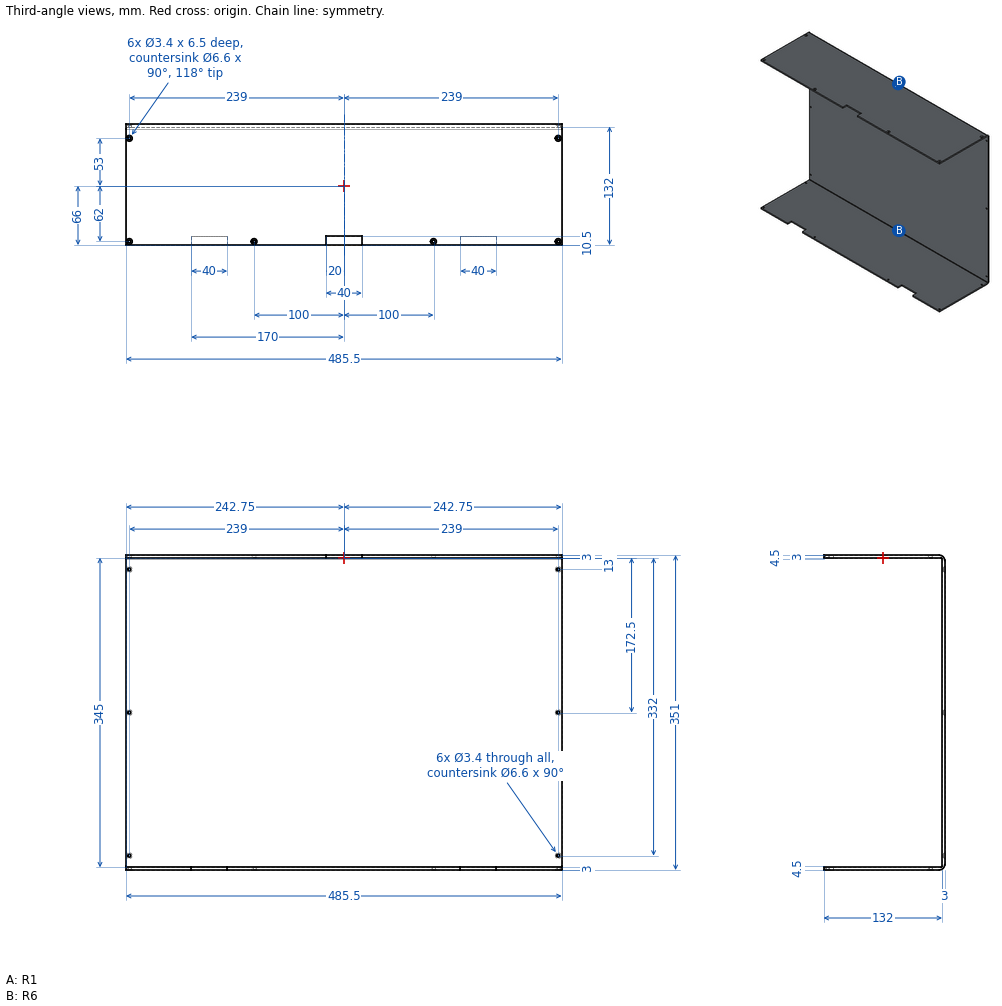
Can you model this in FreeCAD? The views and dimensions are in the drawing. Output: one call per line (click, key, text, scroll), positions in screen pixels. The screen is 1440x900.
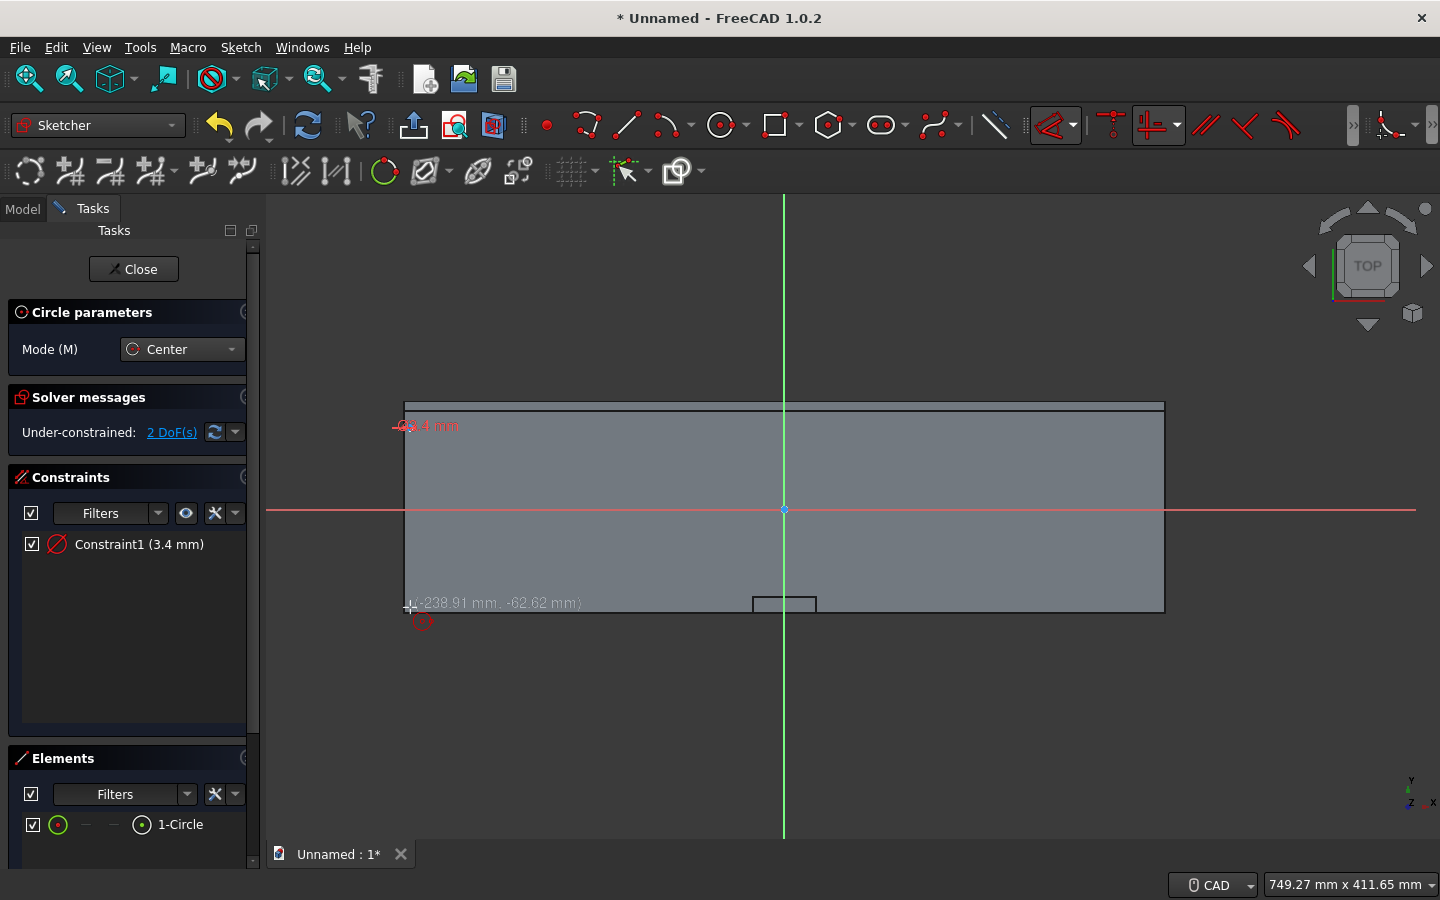
click(410, 607)
move(412, 605)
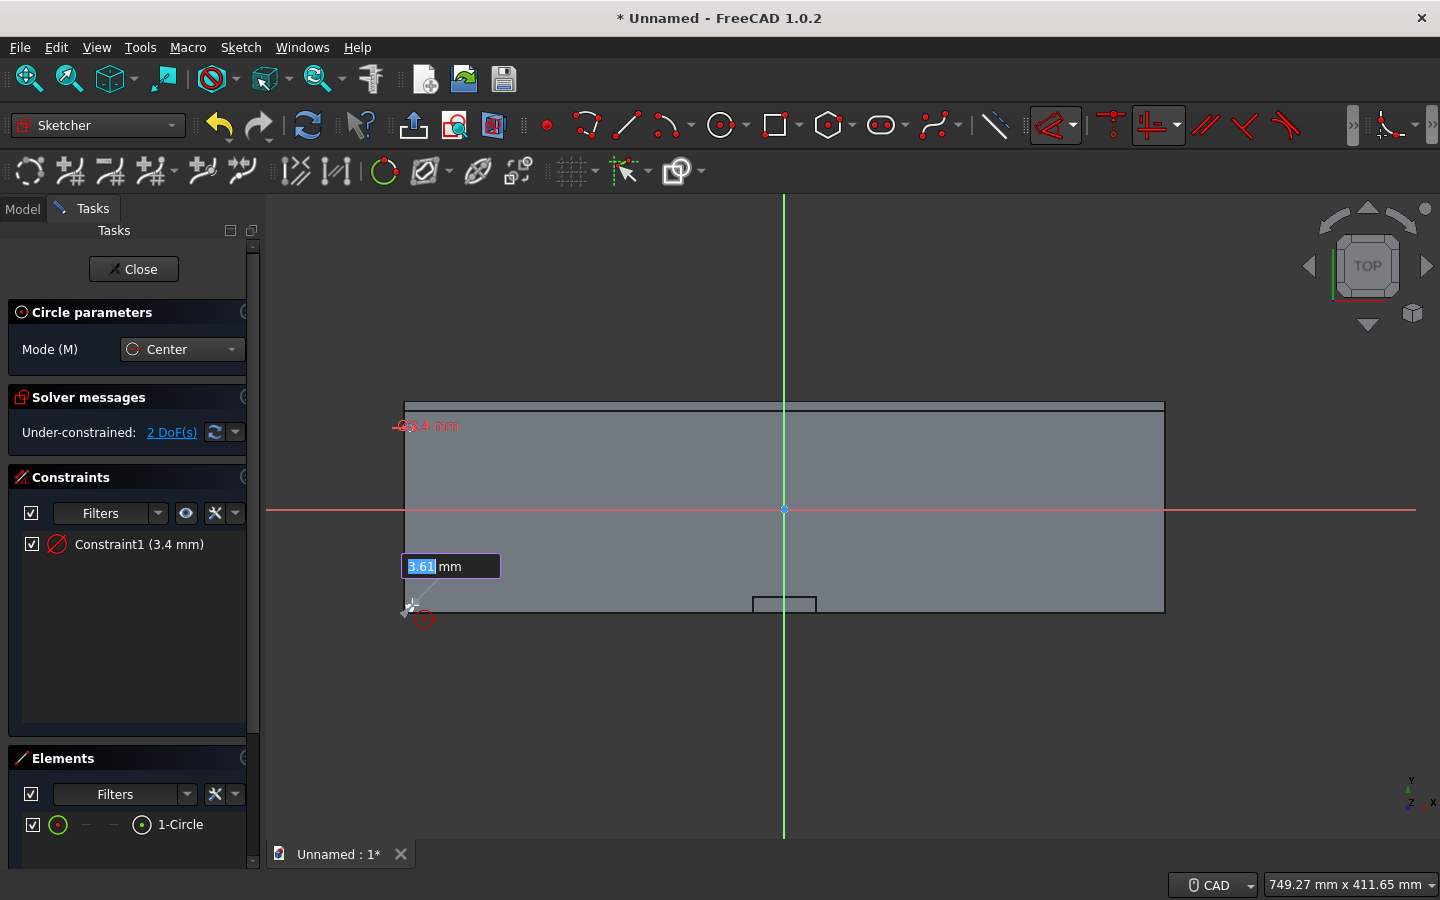
text(3.4)
key(Return)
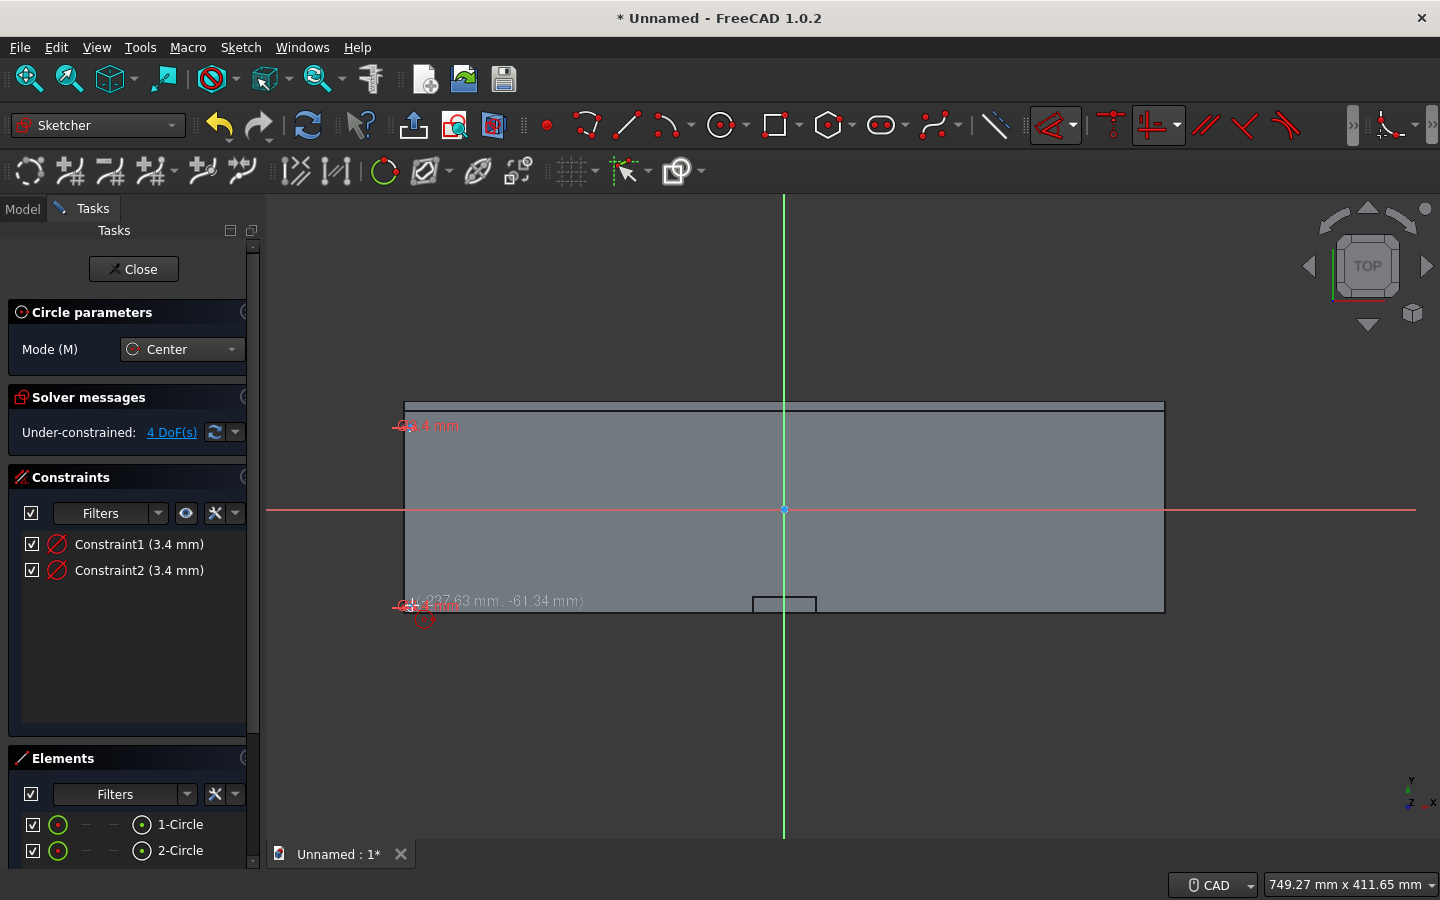
scroll(628, 607, up, 11)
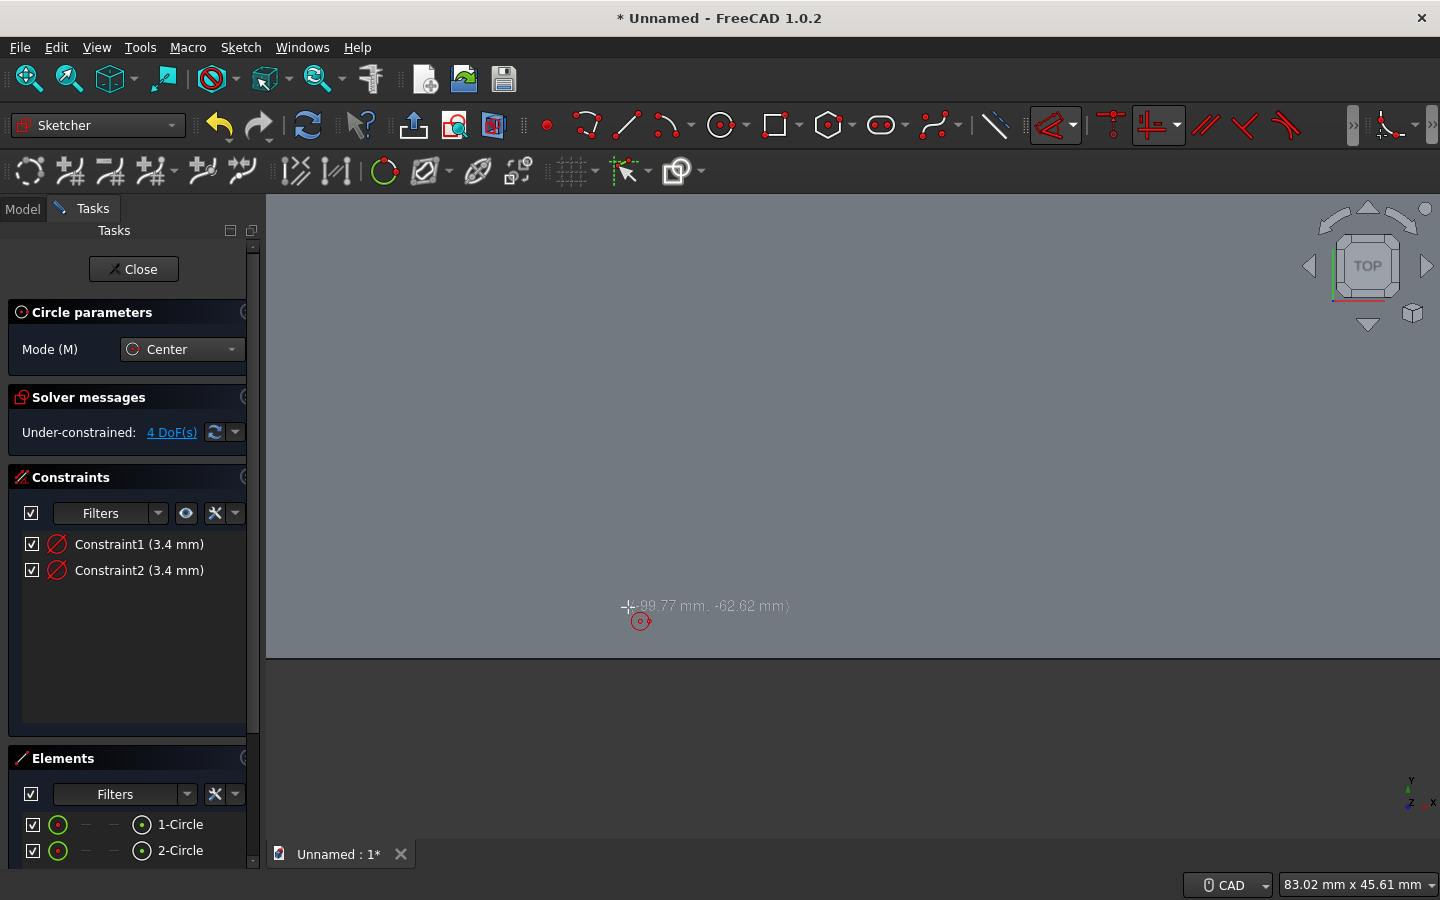
scroll(628, 607, down, 11)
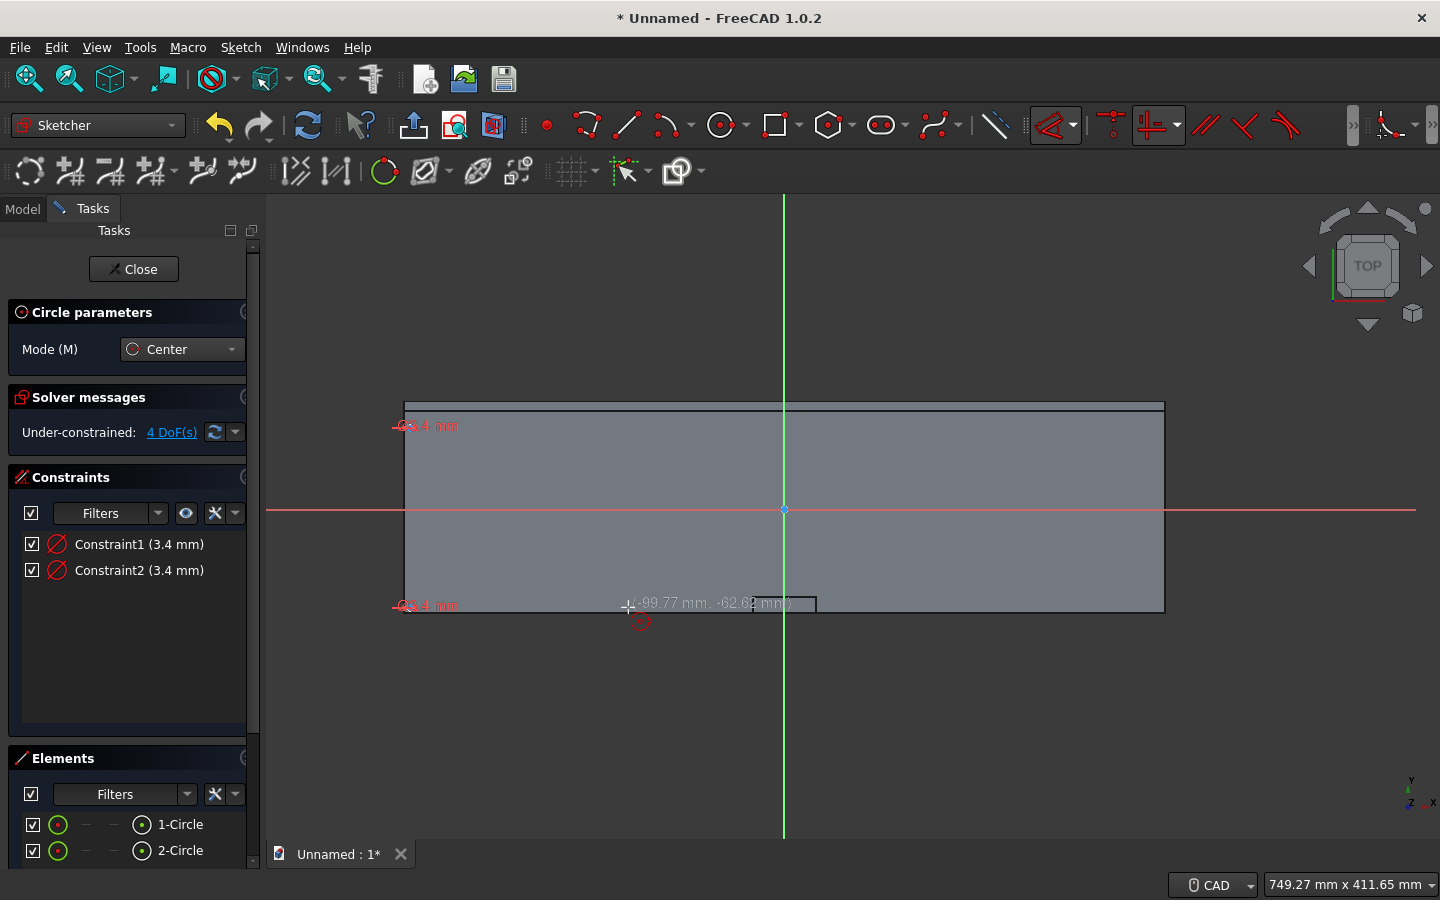
click(628, 607)
move(630, 605)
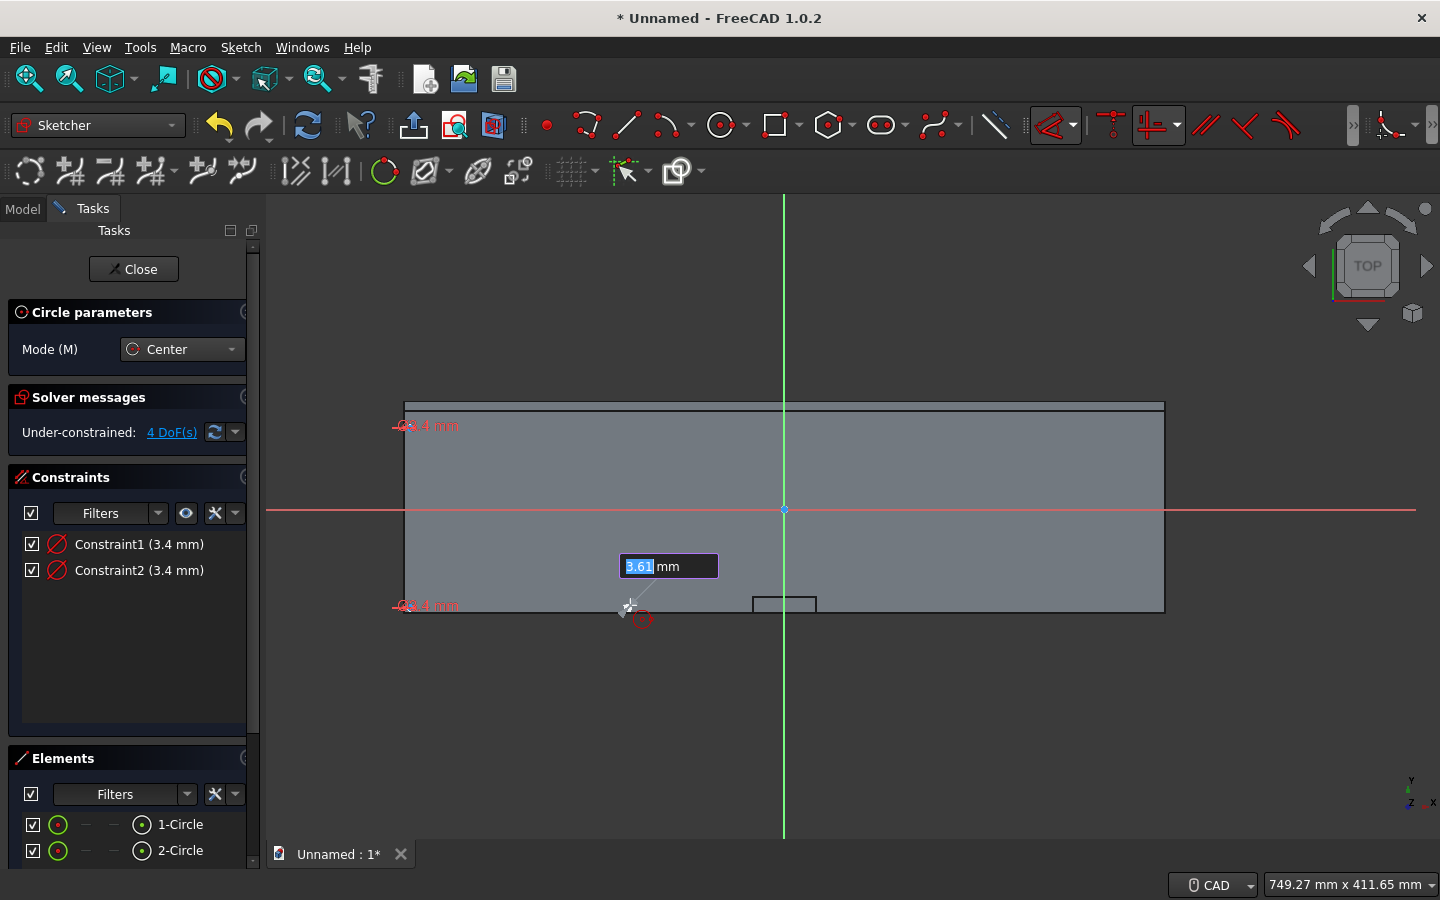
text(3.4)
key(Return)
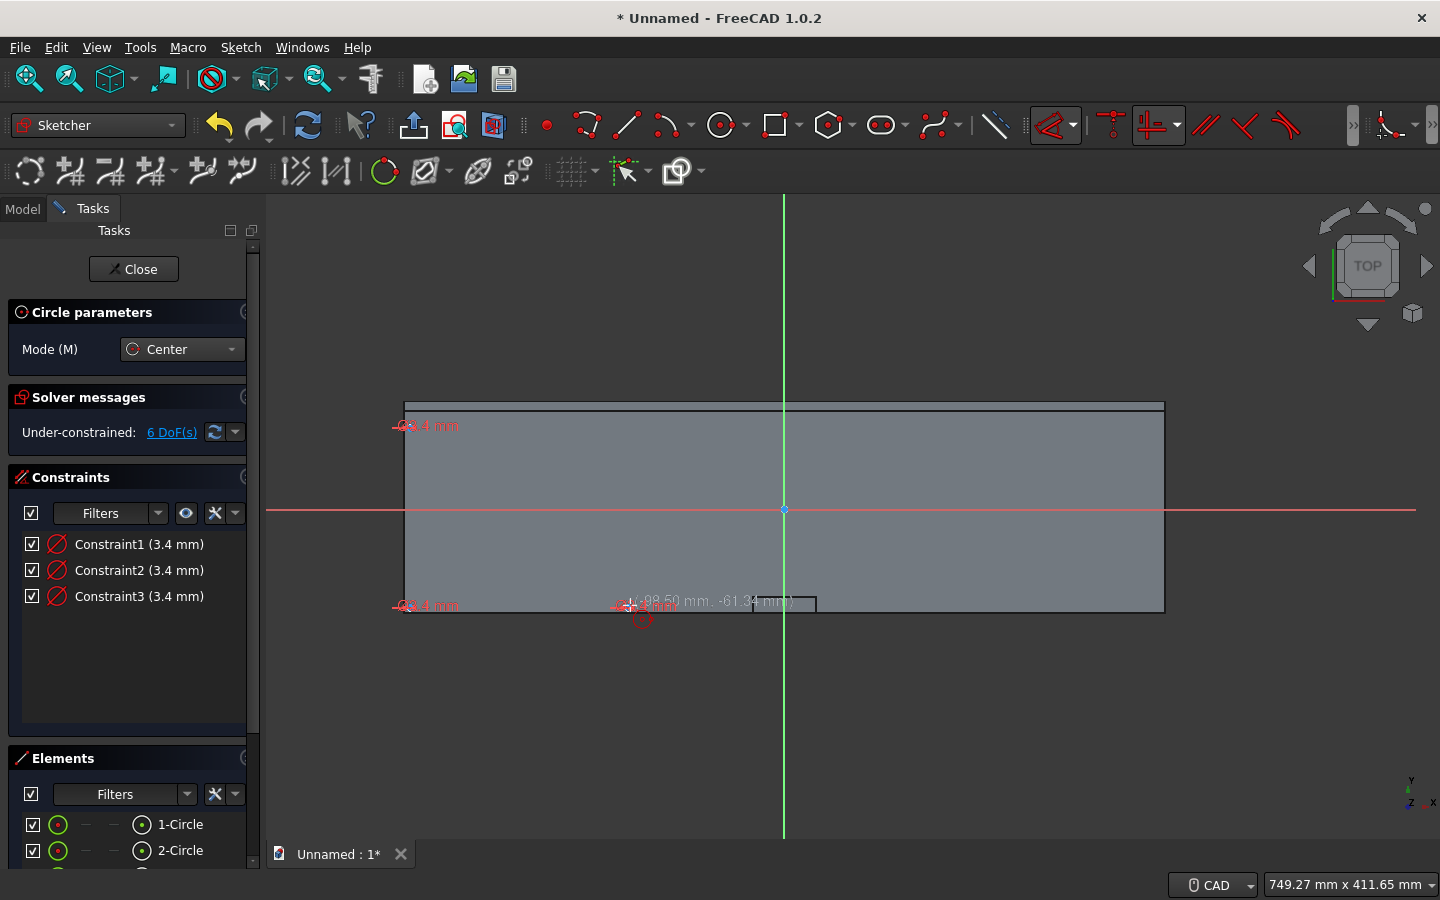
scroll(941, 607, up, 11)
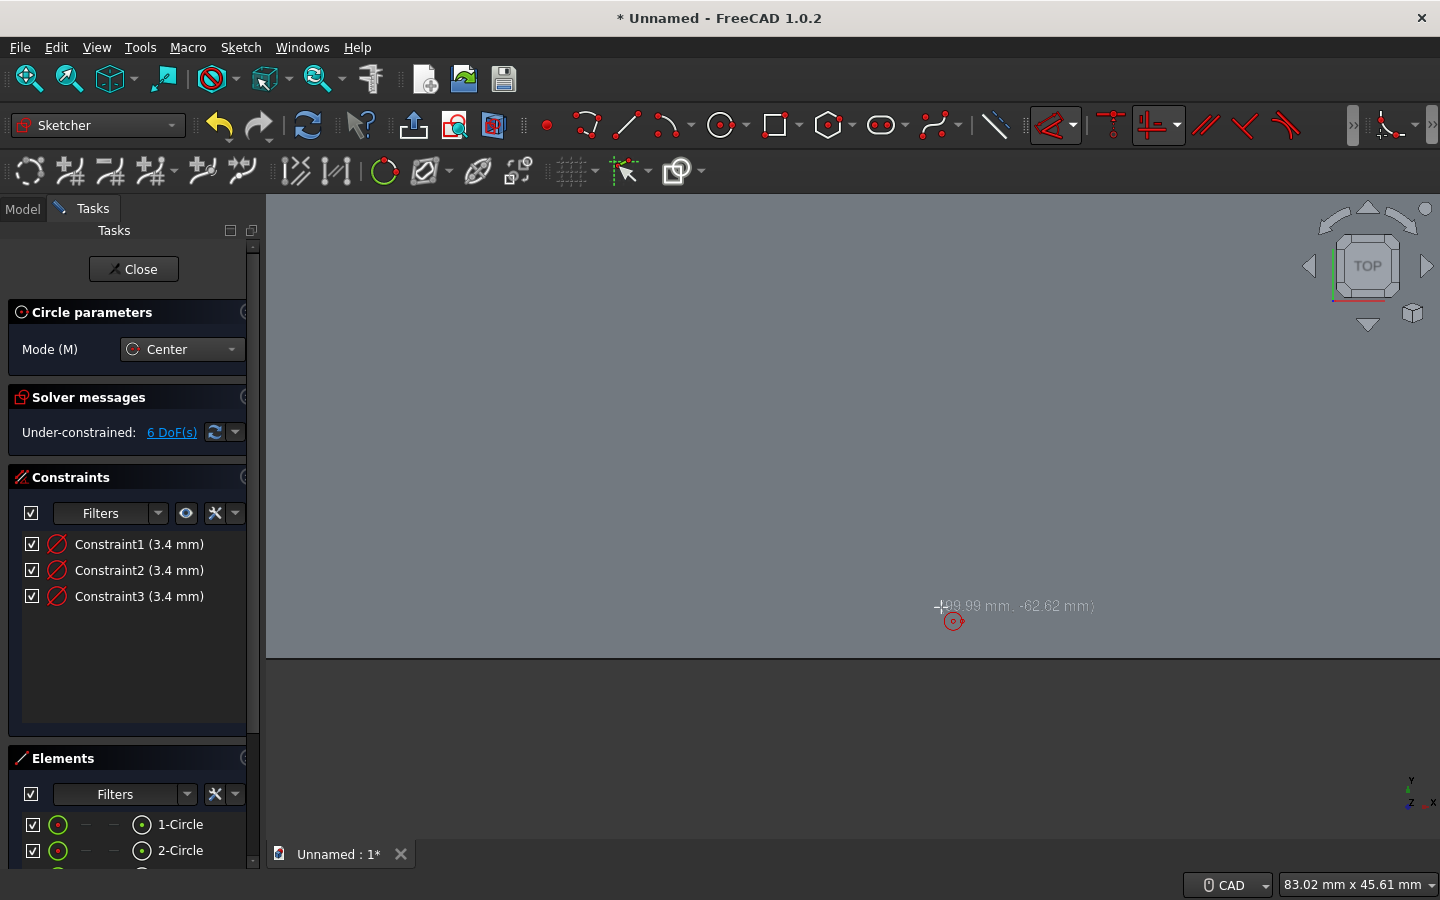
scroll(942, 607, down, 11)